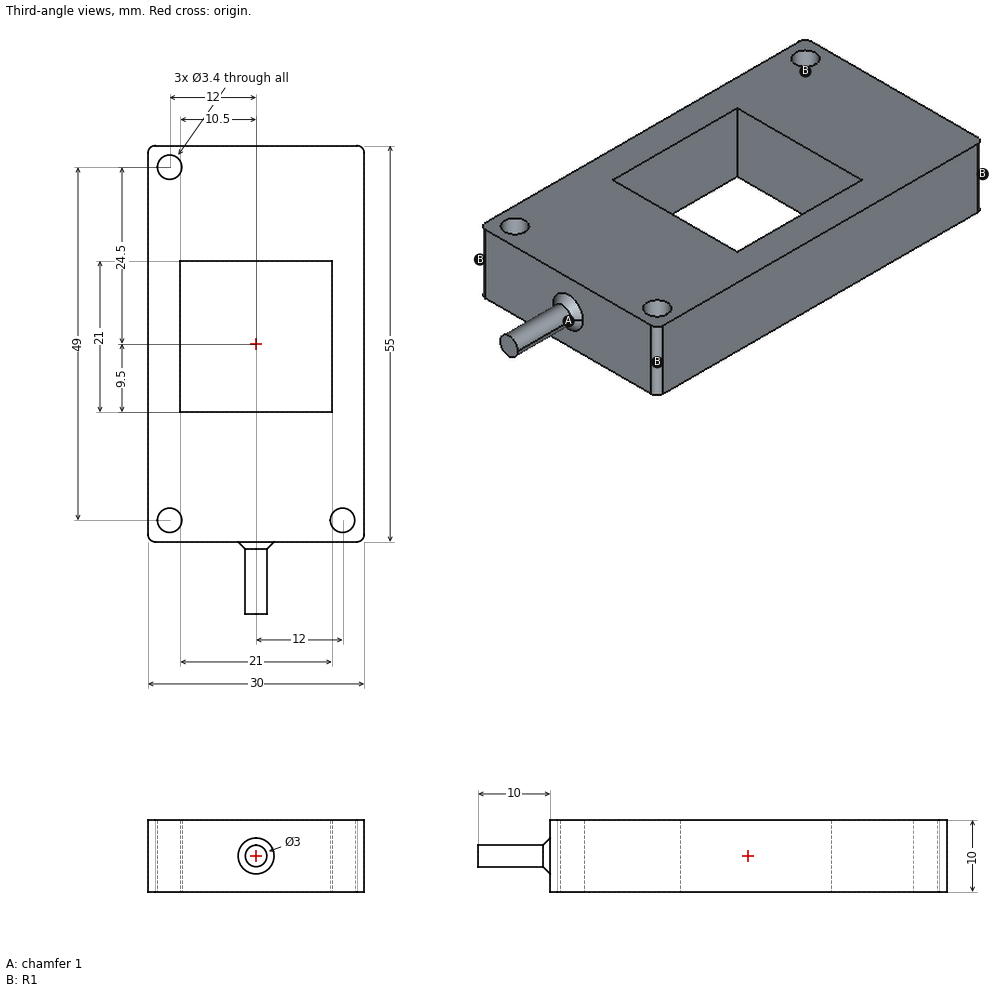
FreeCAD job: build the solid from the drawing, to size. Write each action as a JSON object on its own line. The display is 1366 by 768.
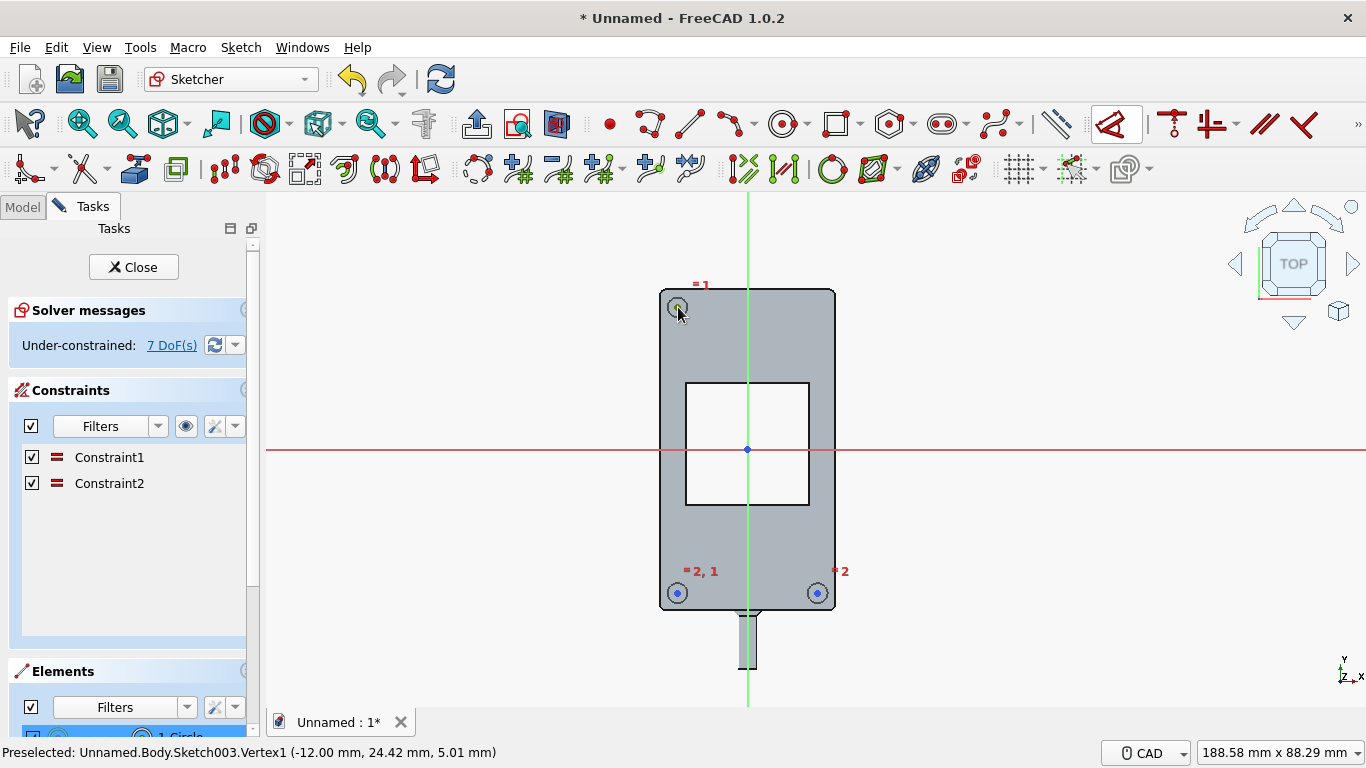
{"action": "left_click", "coordinate": [678, 593]}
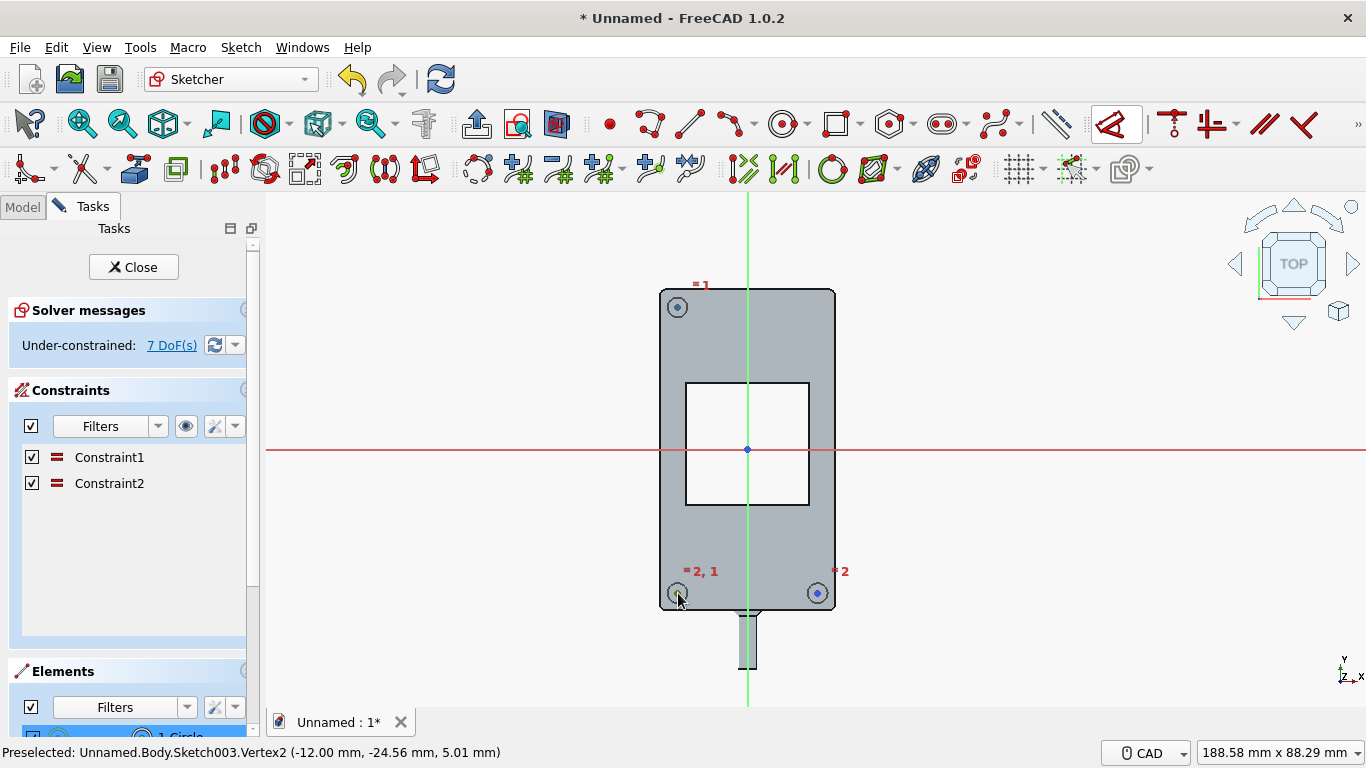
{"action": "key", "text": "v"}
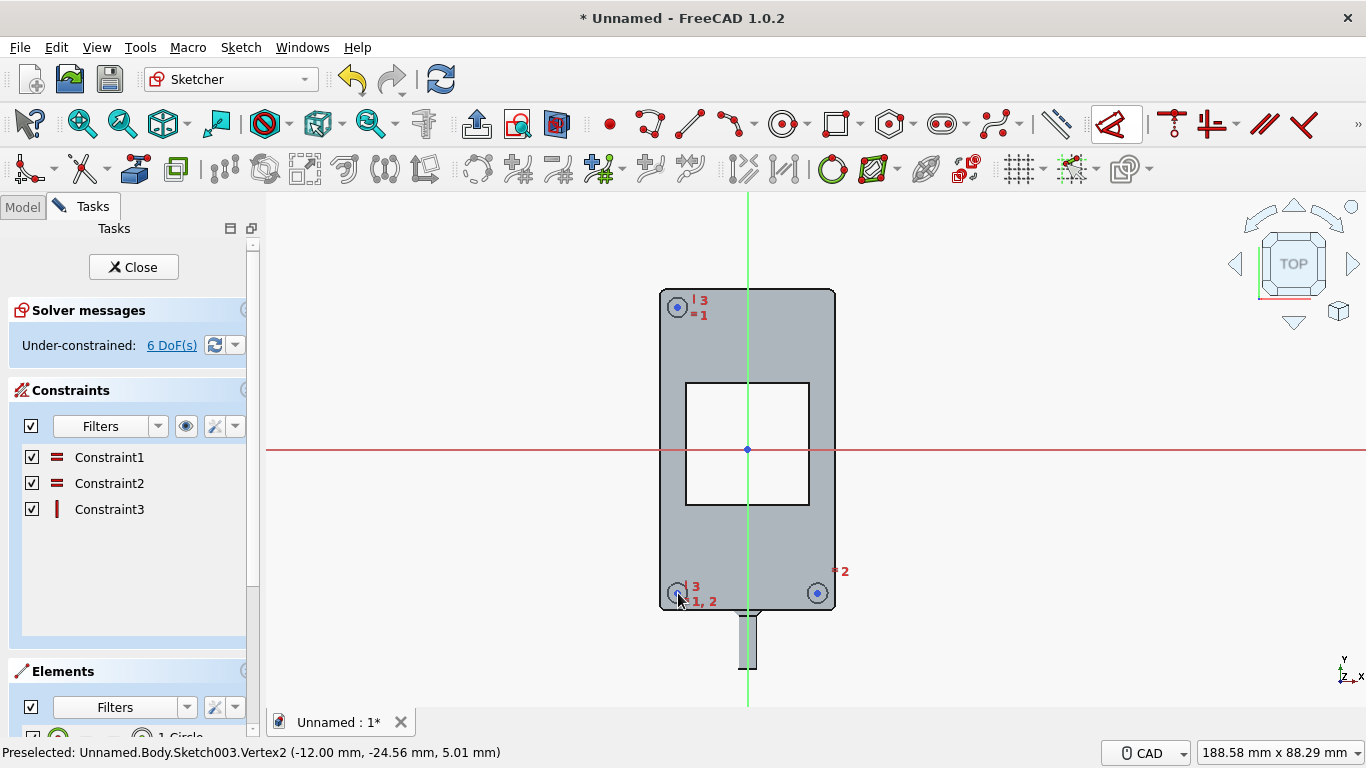
{"action": "left_click", "coordinate": [678, 593]}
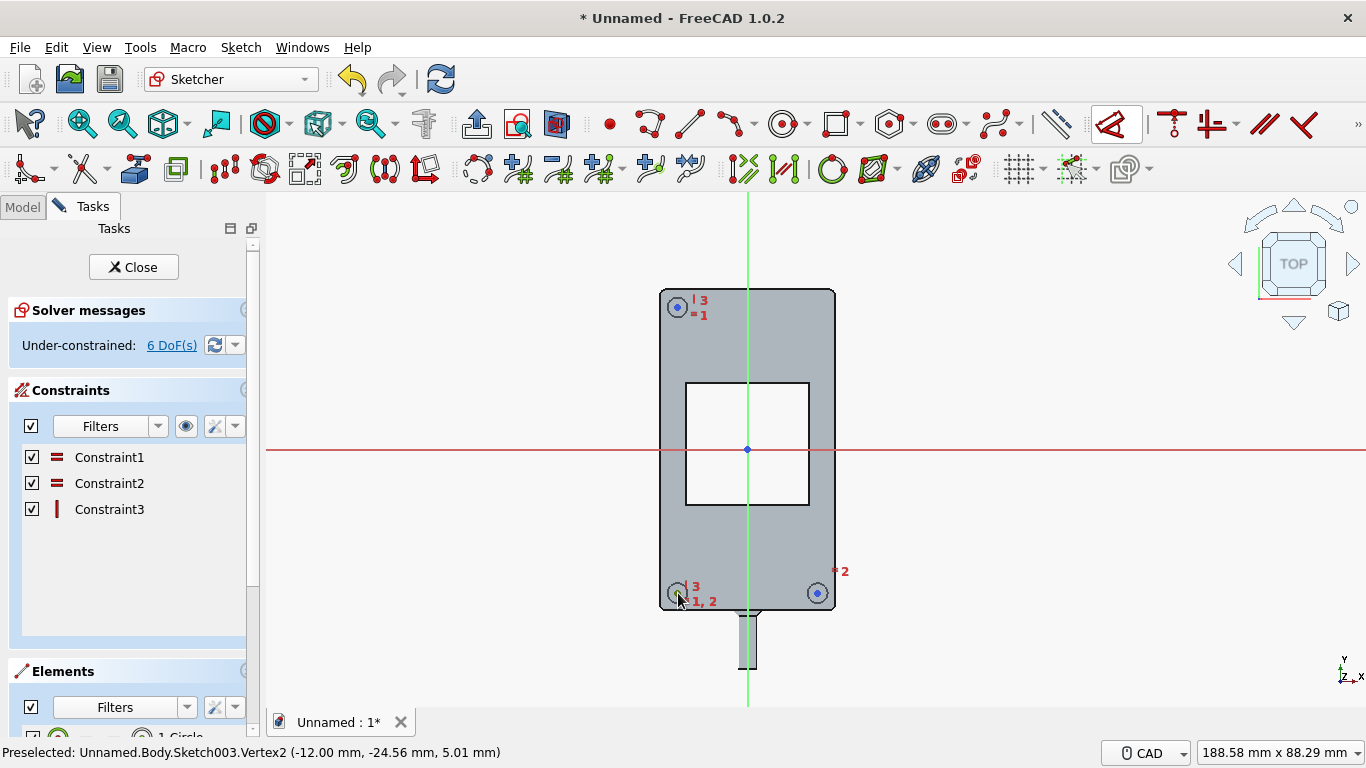
{"action": "left_click", "coordinate": [818, 593]}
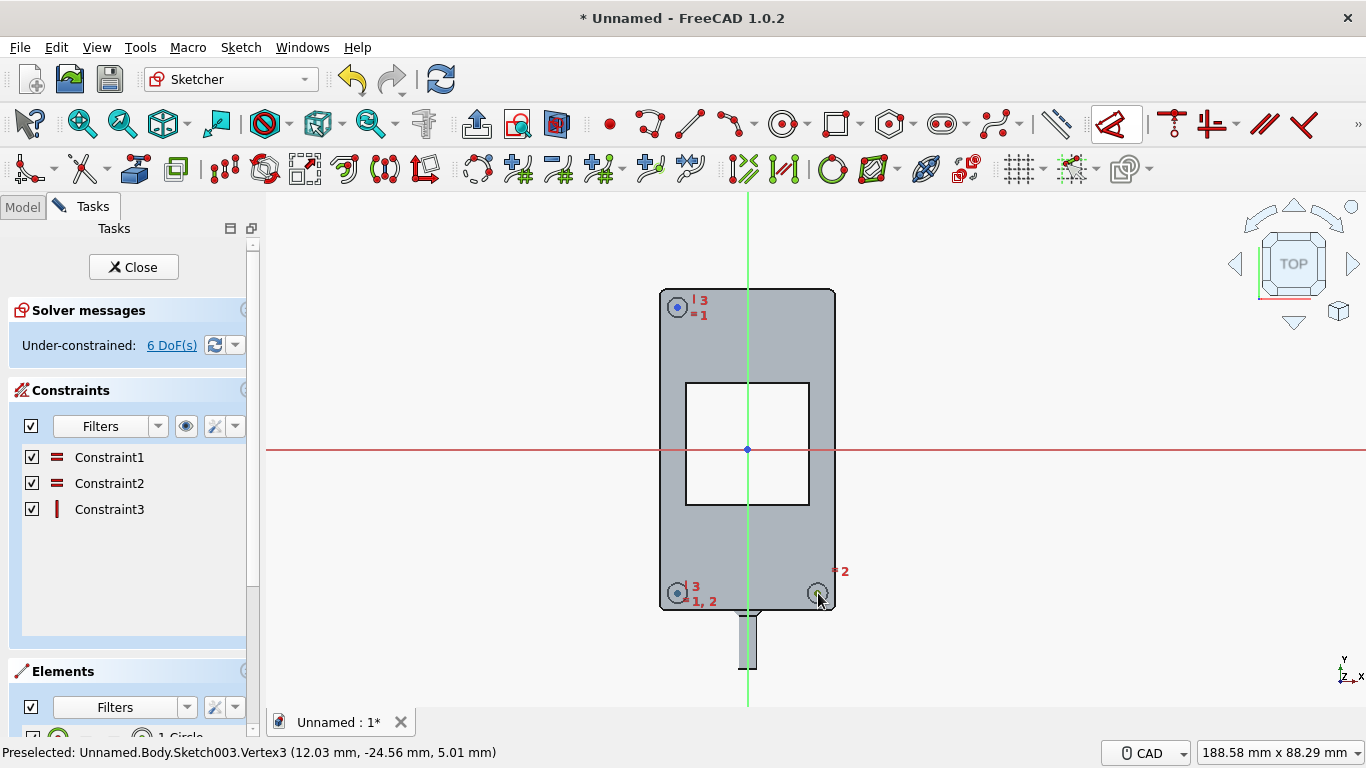
{"action": "key", "text": "h"}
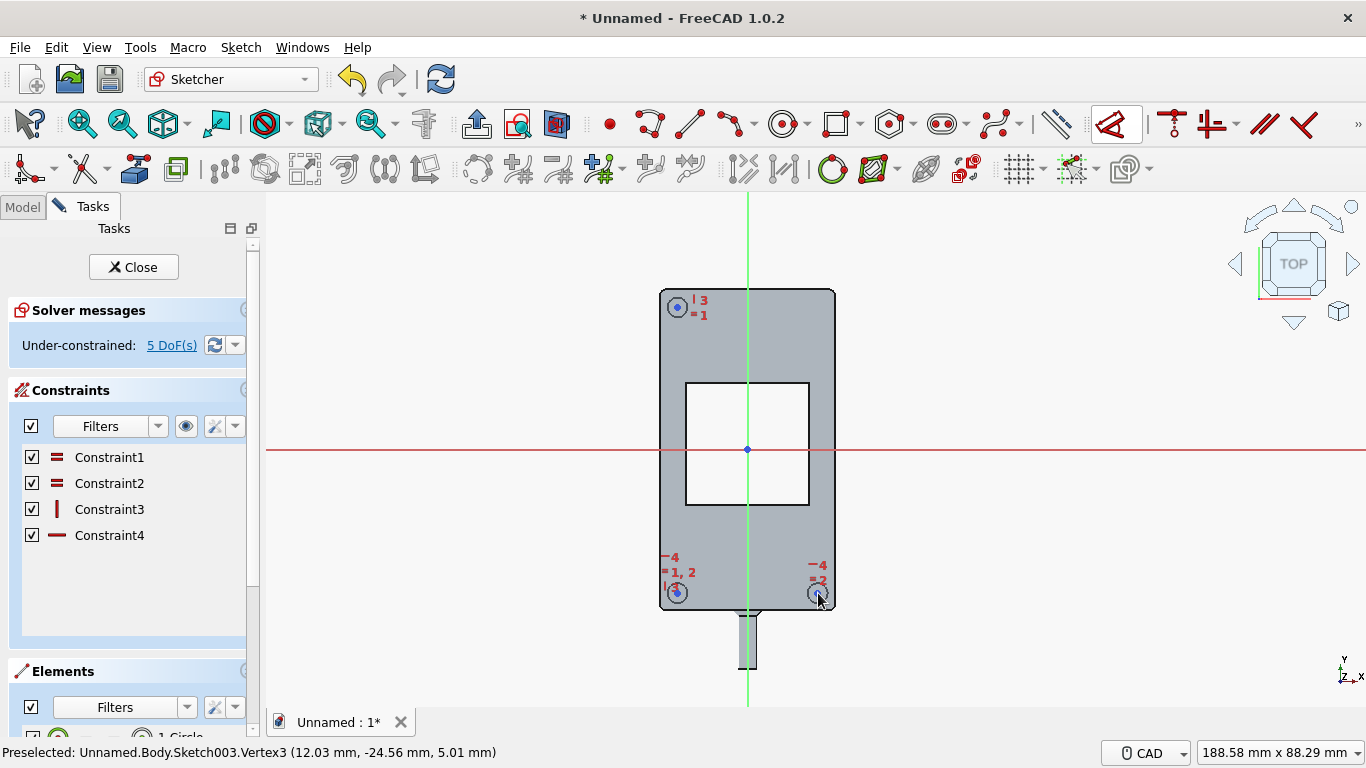
{"action": "key", "text": "d"}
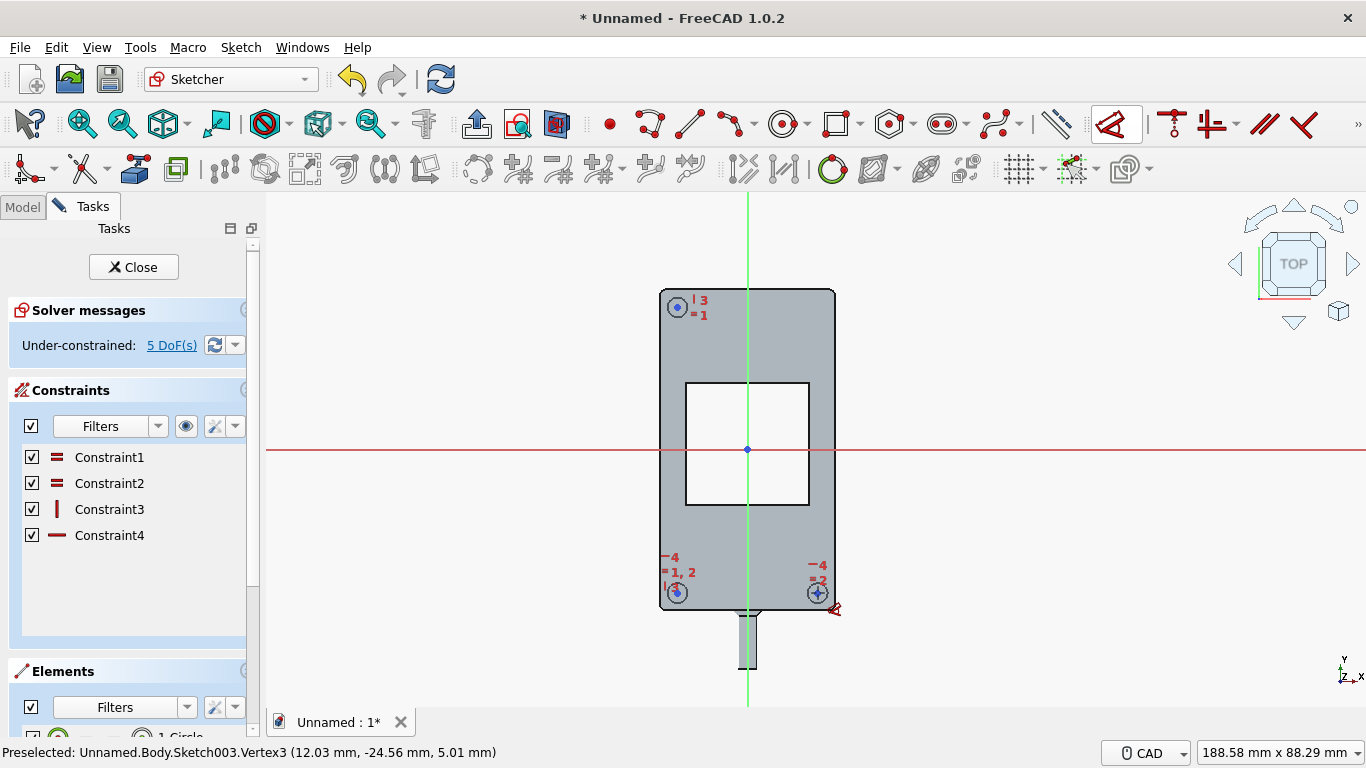
{"action": "scroll", "coordinate": [684, 300], "scroll_direction": "up", "scroll_amount": 4}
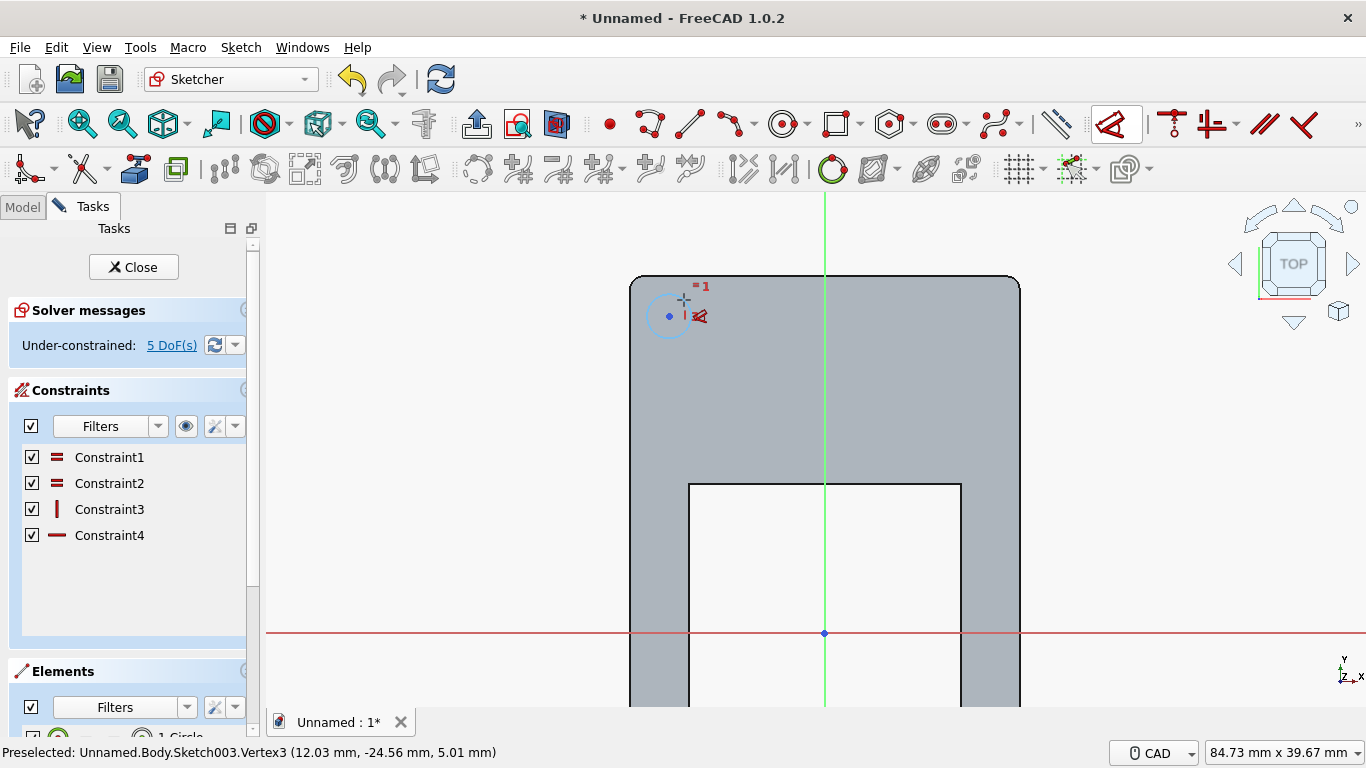
{"action": "left_click", "coordinate": [685, 301]}
{"action": "left_click", "coordinate": [708, 279]}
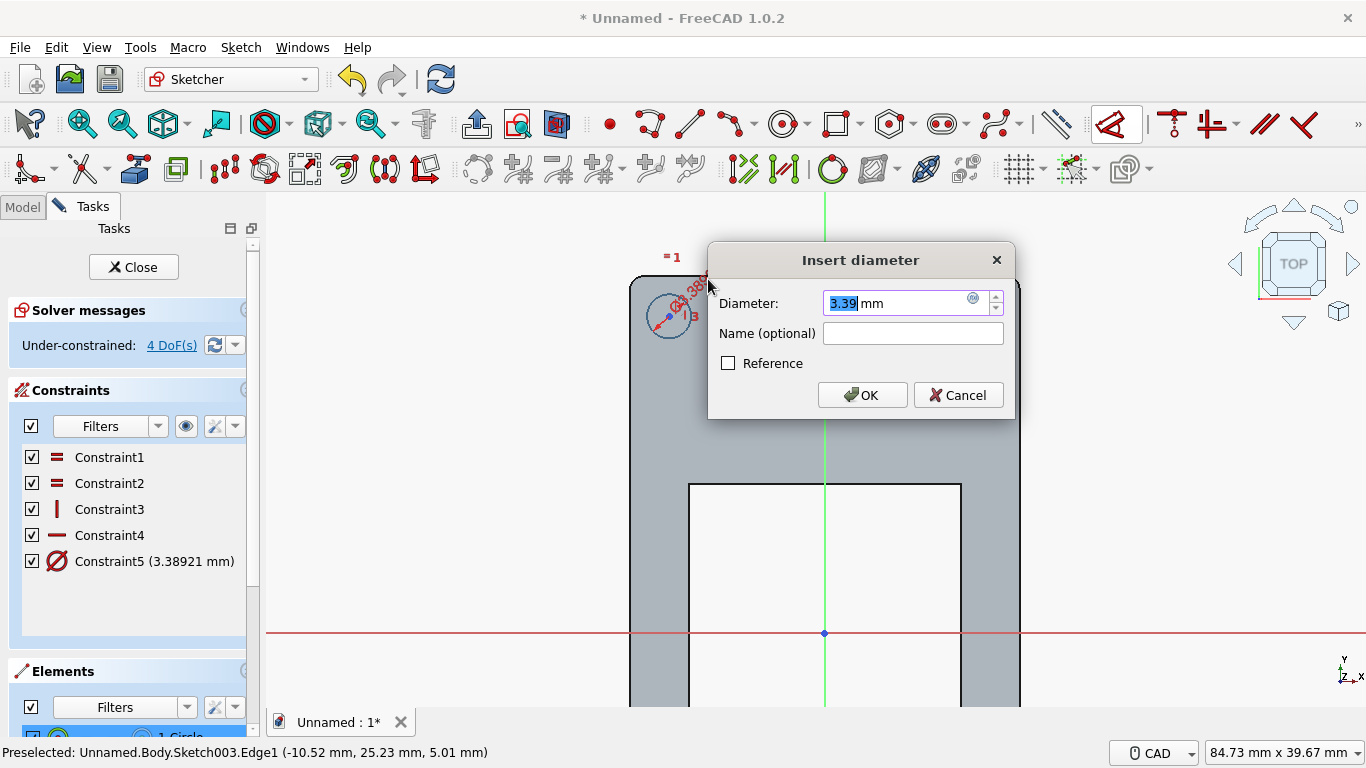
{"action": "type", "text": "3.4"}
{"action": "key", "text": "Return"}